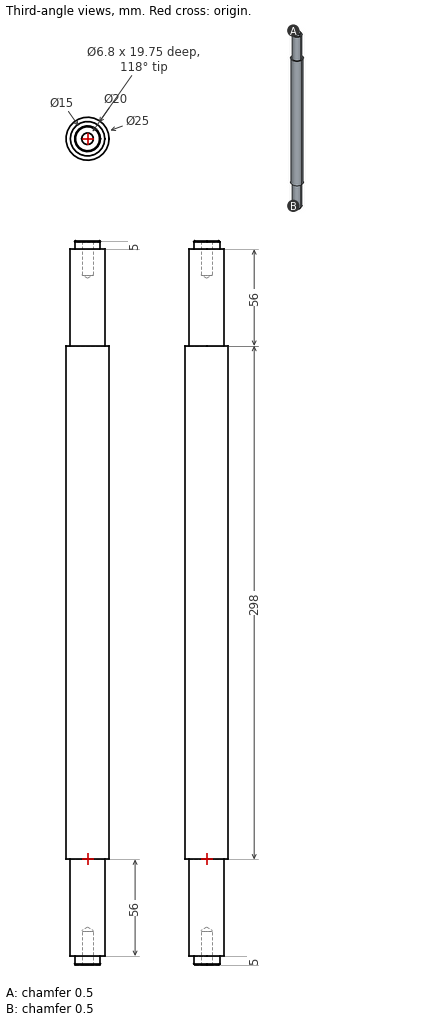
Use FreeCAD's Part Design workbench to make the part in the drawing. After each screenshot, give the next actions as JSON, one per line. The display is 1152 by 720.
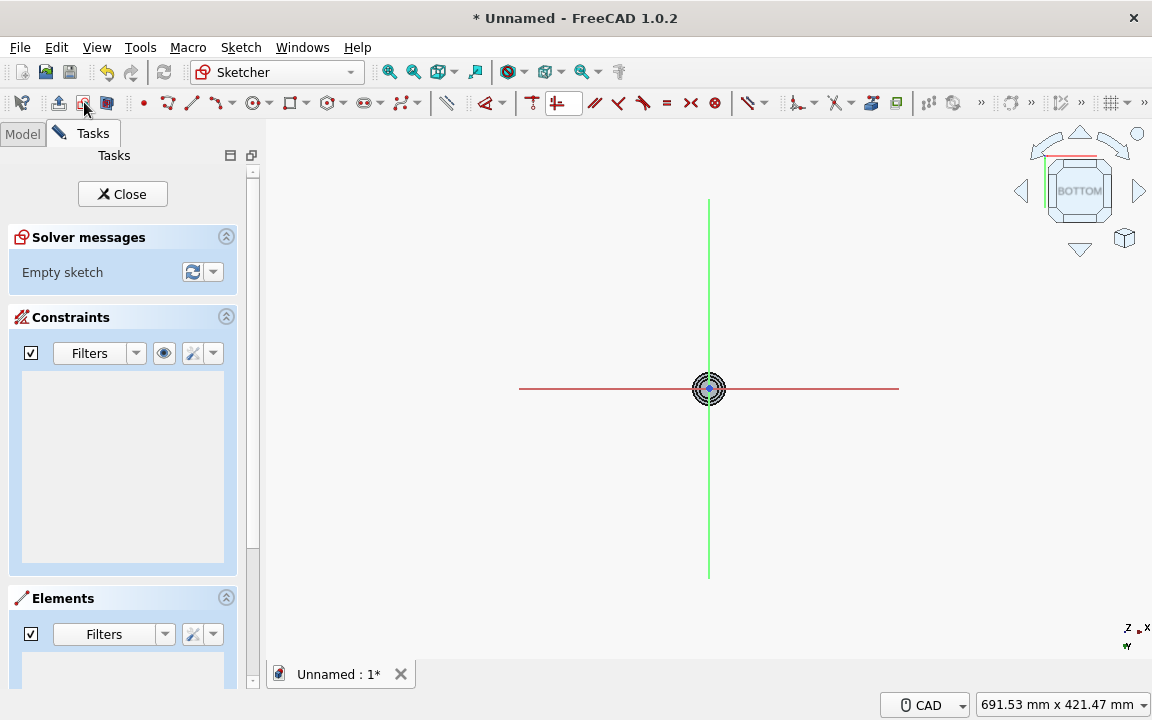
{"action": "scroll", "coordinate": [713, 389], "scroll_direction": "up", "scroll_amount": 15}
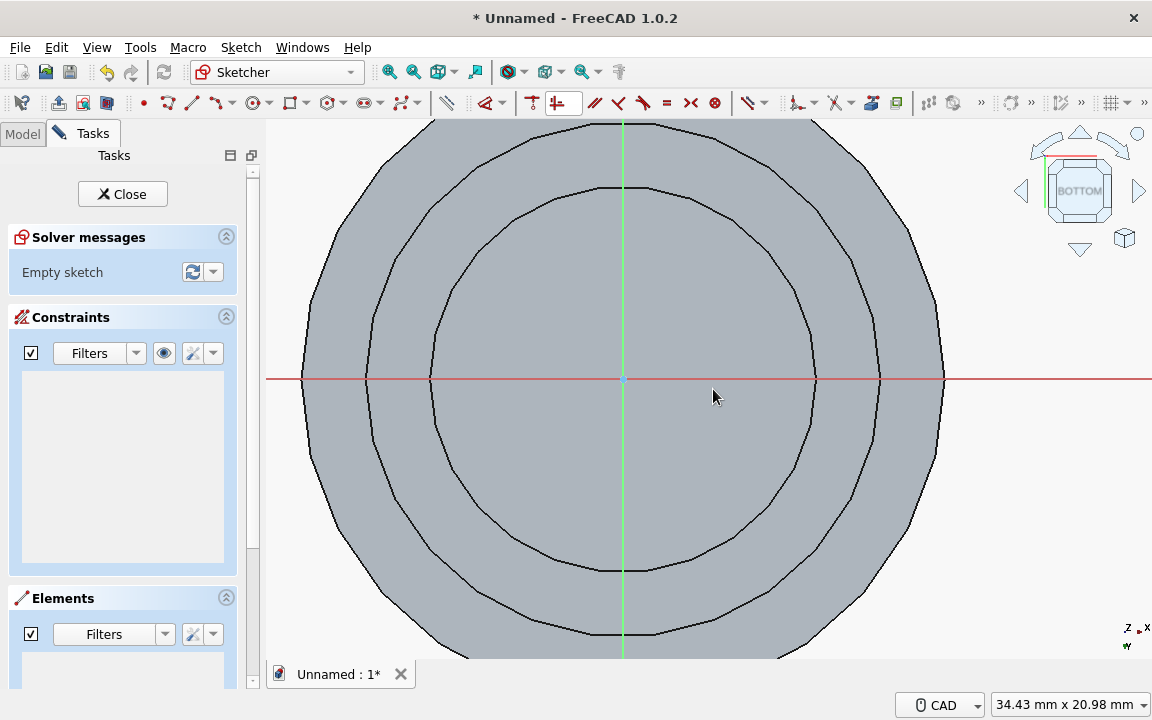
{"action": "scroll", "coordinate": [602, 368], "scroll_direction": "up", "scroll_amount": 3}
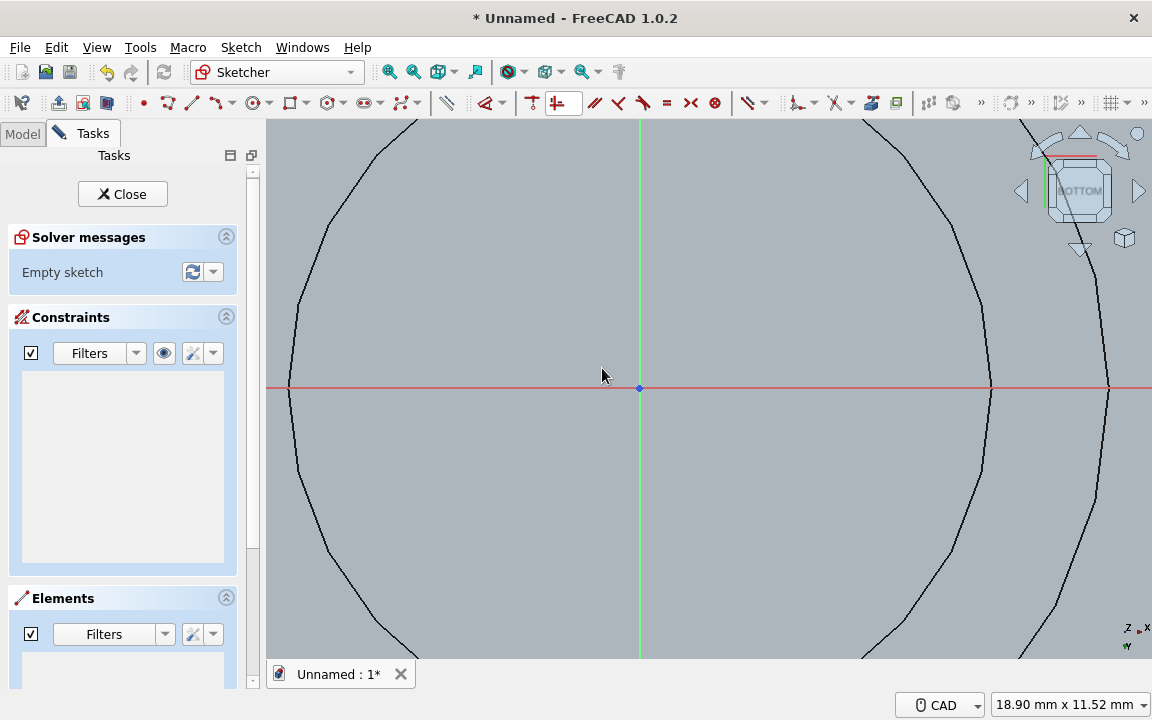
{"action": "left_click", "coordinate": [254, 104]}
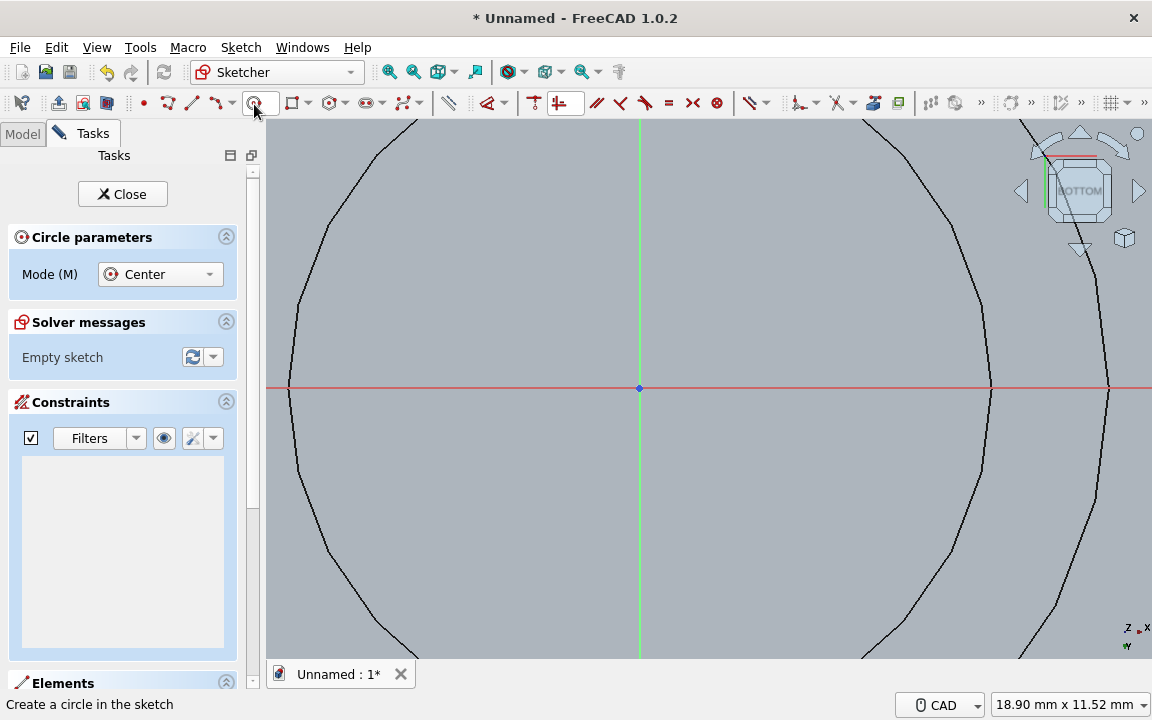
{"action": "left_click", "coordinate": [640, 388]}
{"action": "left_click", "coordinate": [753, 276]}
{"action": "key", "text": "Escape"}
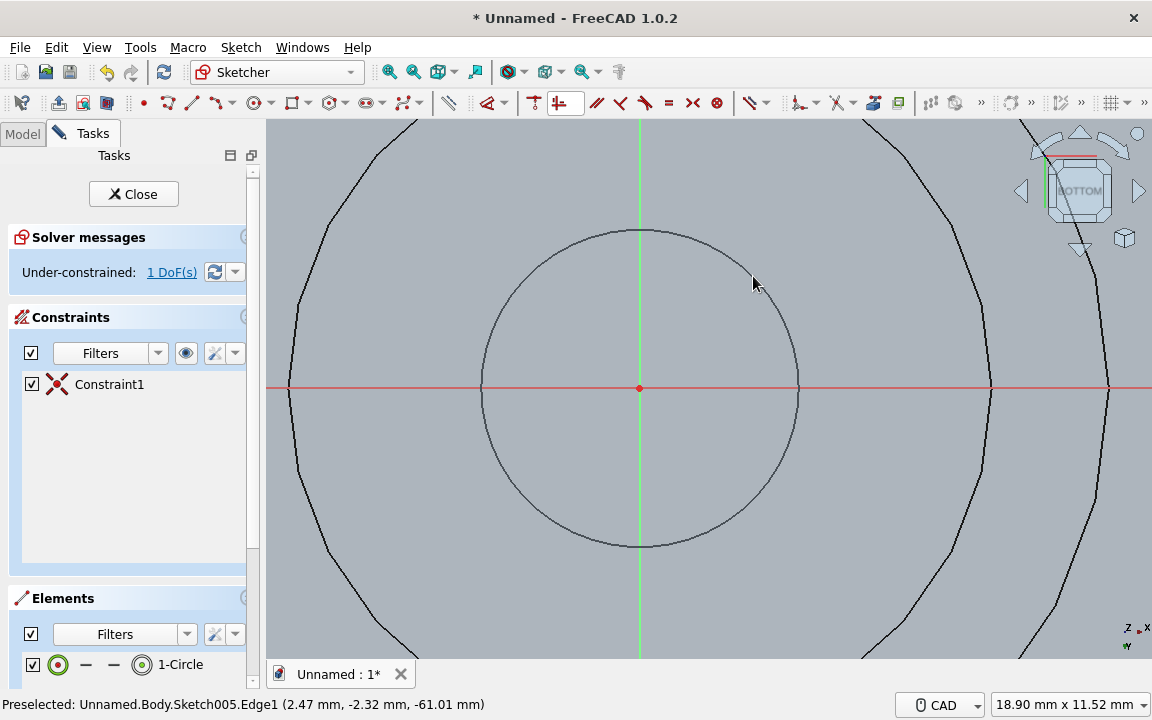
{"action": "left_click", "coordinate": [488, 104]}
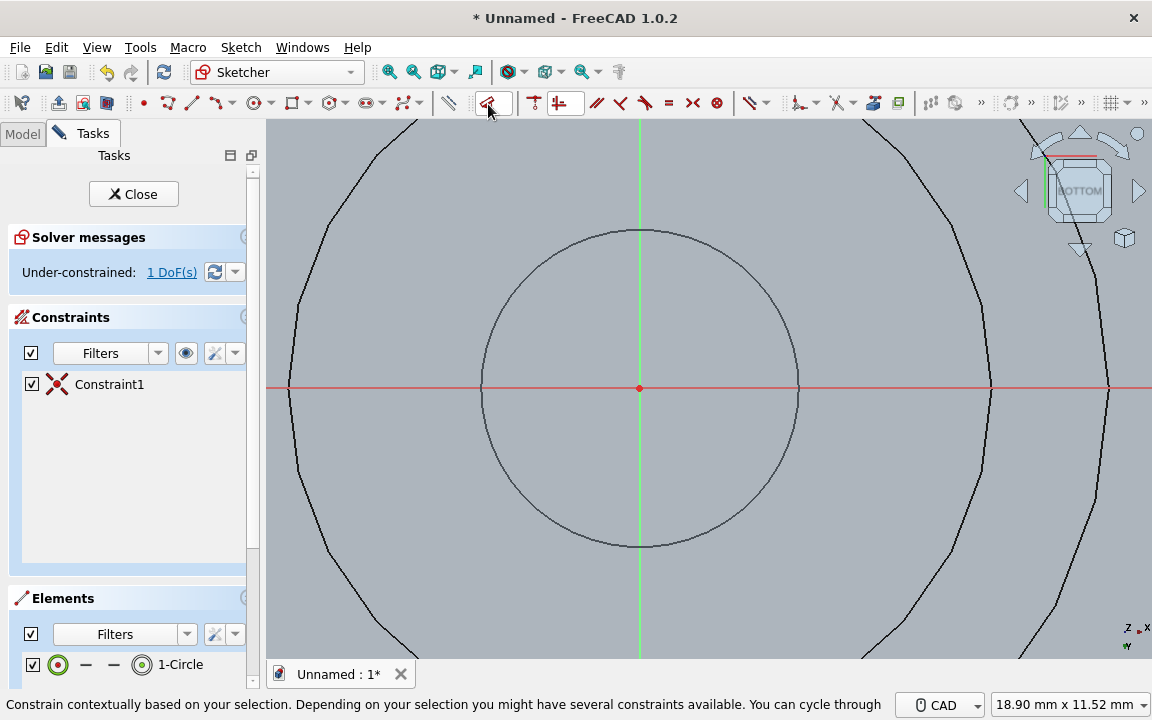
{"action": "left_click", "coordinate": [752, 276]}
{"action": "left_click", "coordinate": [775, 253]}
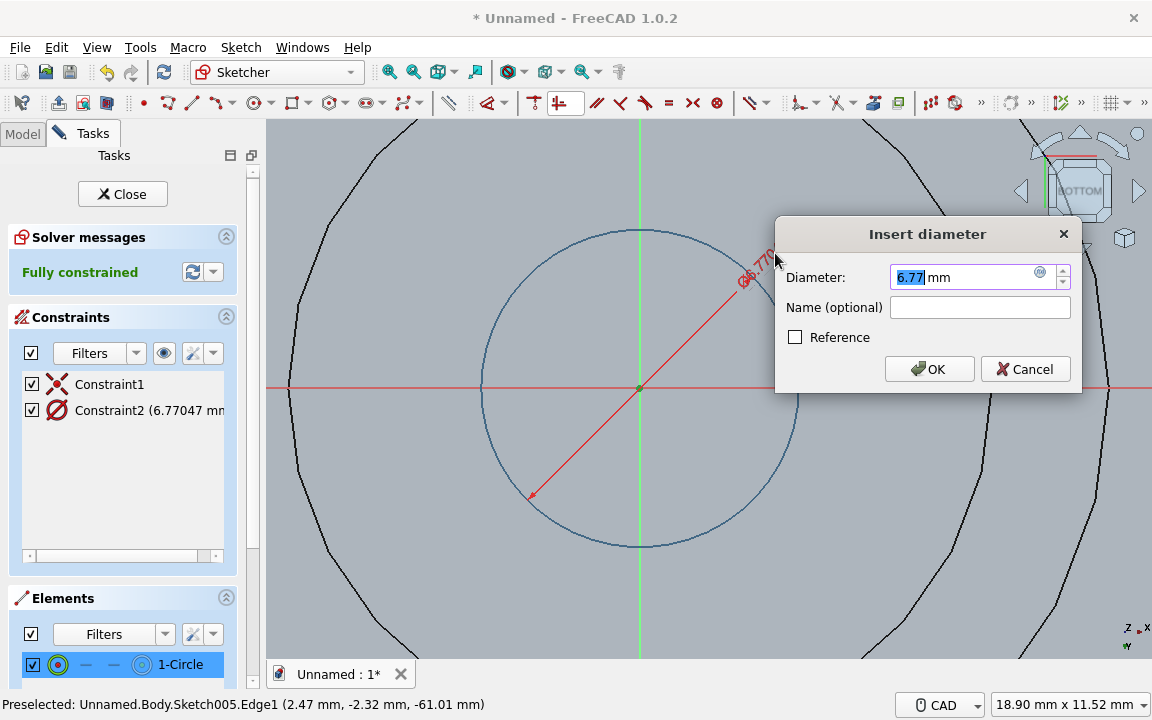
{"action": "type", "text": "6.8"}
{"action": "key", "text": "Return"}
{"action": "key", "text": "Escape"}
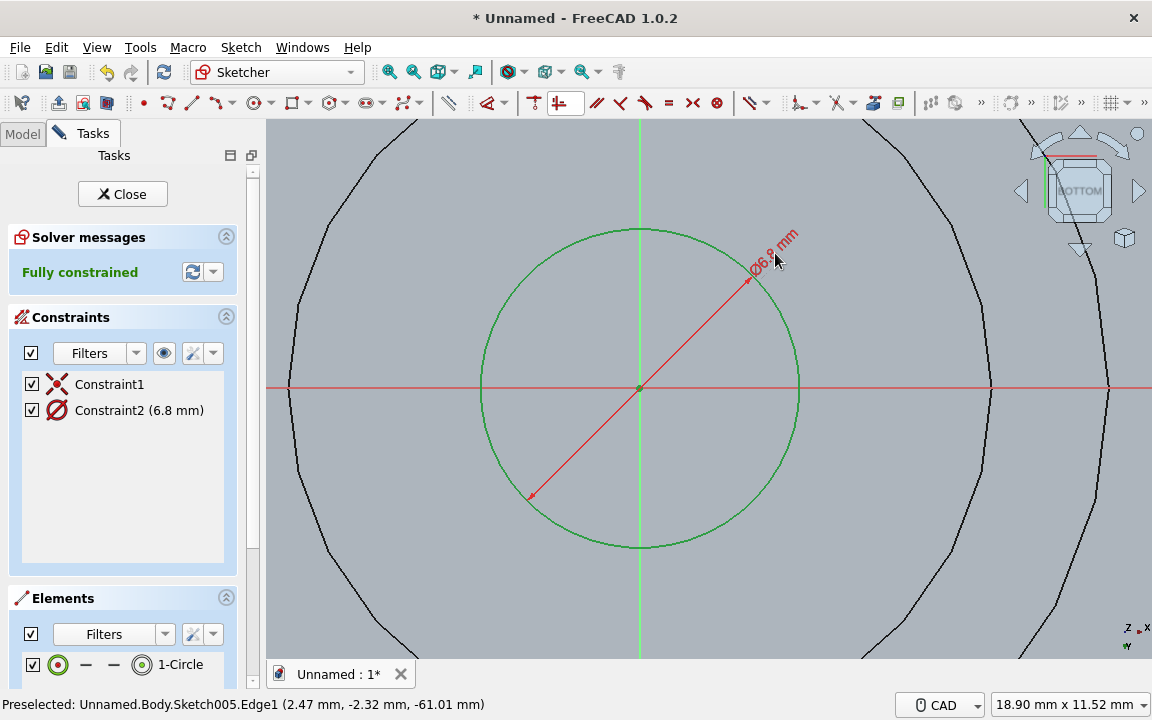
{"action": "left_click", "coordinate": [123, 194]}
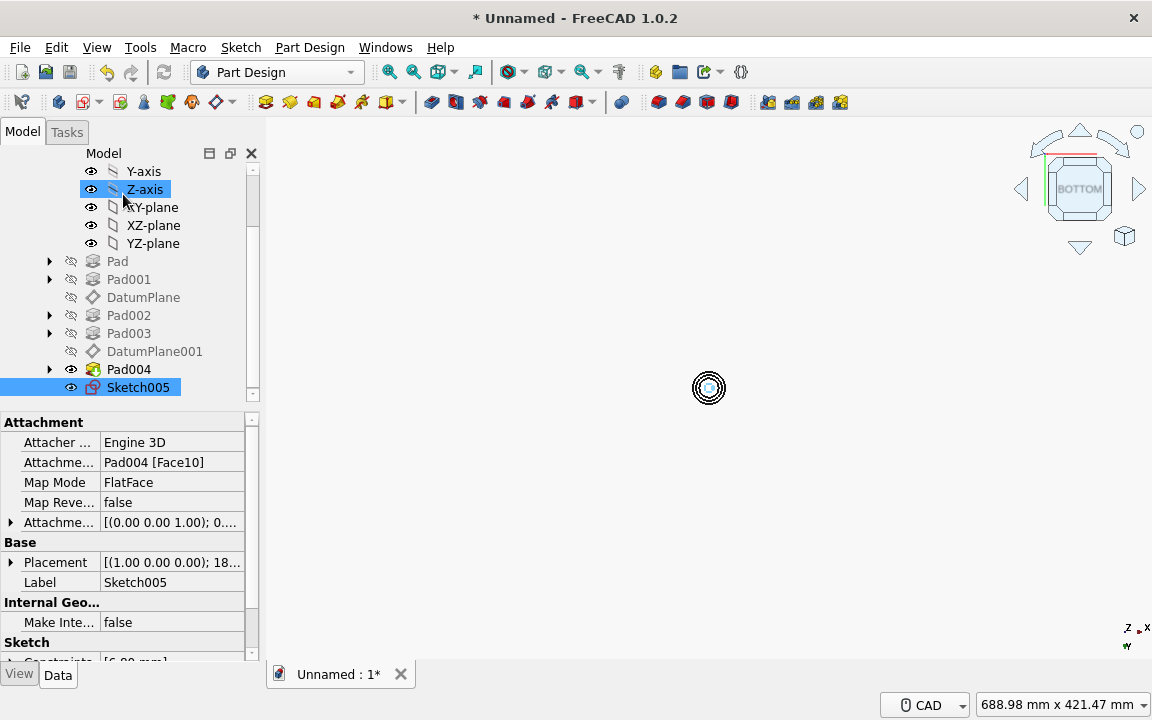
{"action": "left_click", "coordinate": [456, 102]}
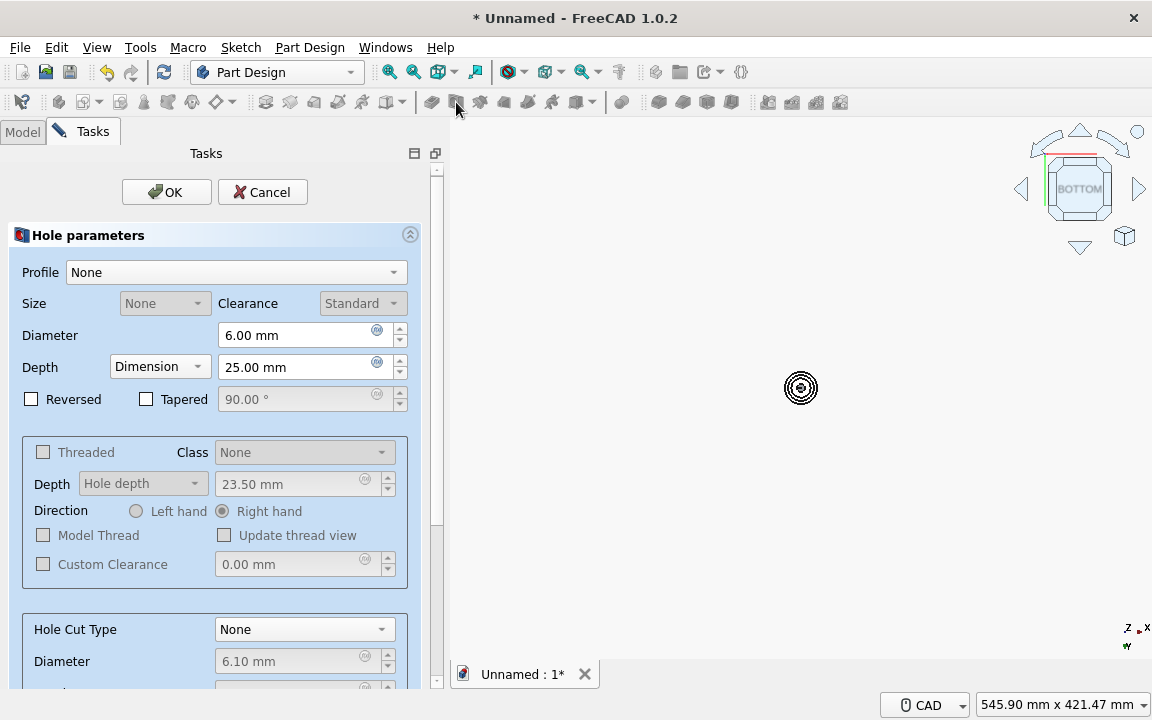
{"action": "triple_click", "coordinate": [305, 335]}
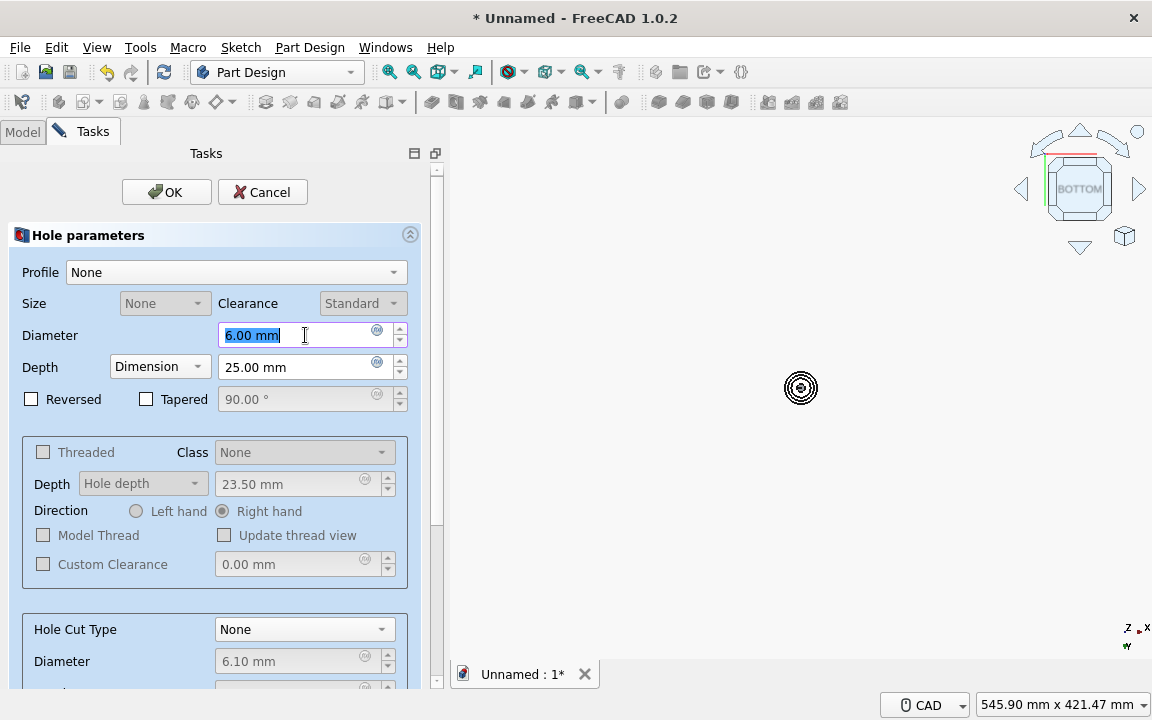
{"action": "type", "text": "6.8"}
{"action": "key", "text": "Tab"}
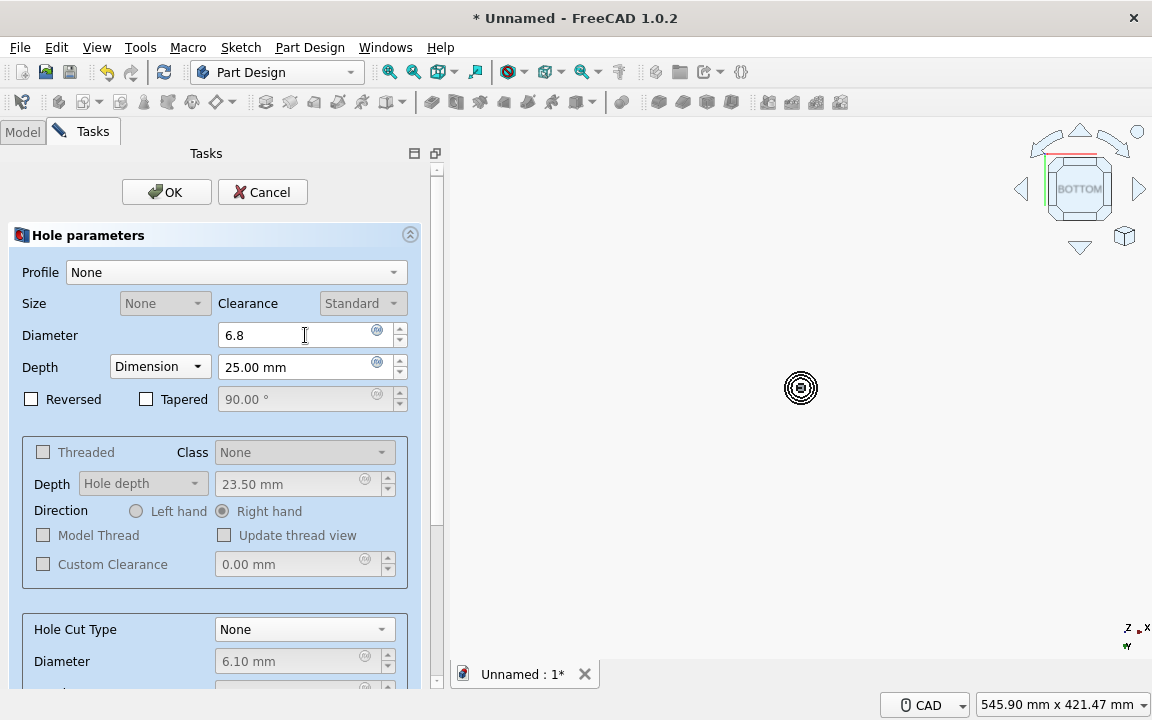
{"action": "triple_click", "coordinate": [305, 367]}